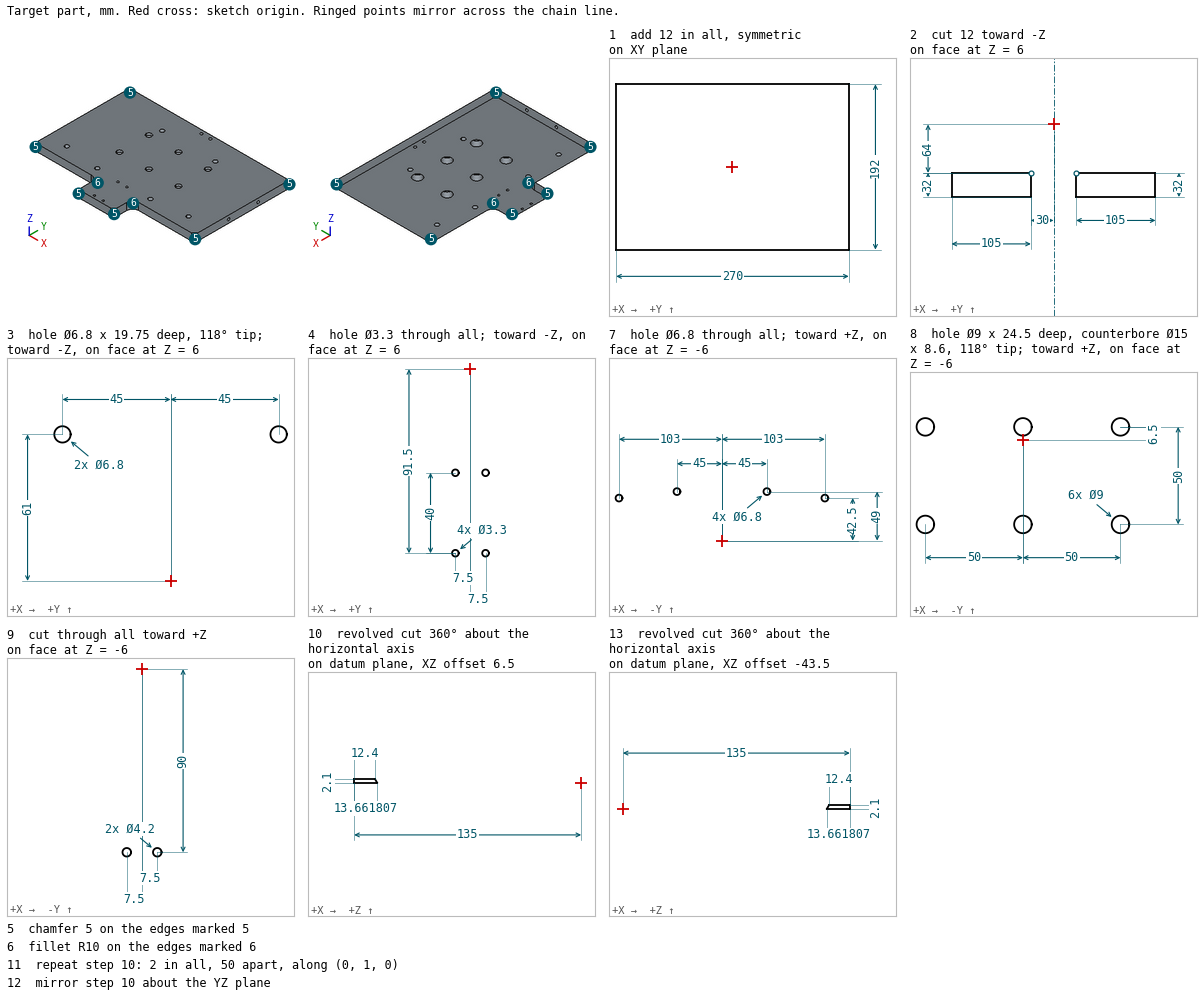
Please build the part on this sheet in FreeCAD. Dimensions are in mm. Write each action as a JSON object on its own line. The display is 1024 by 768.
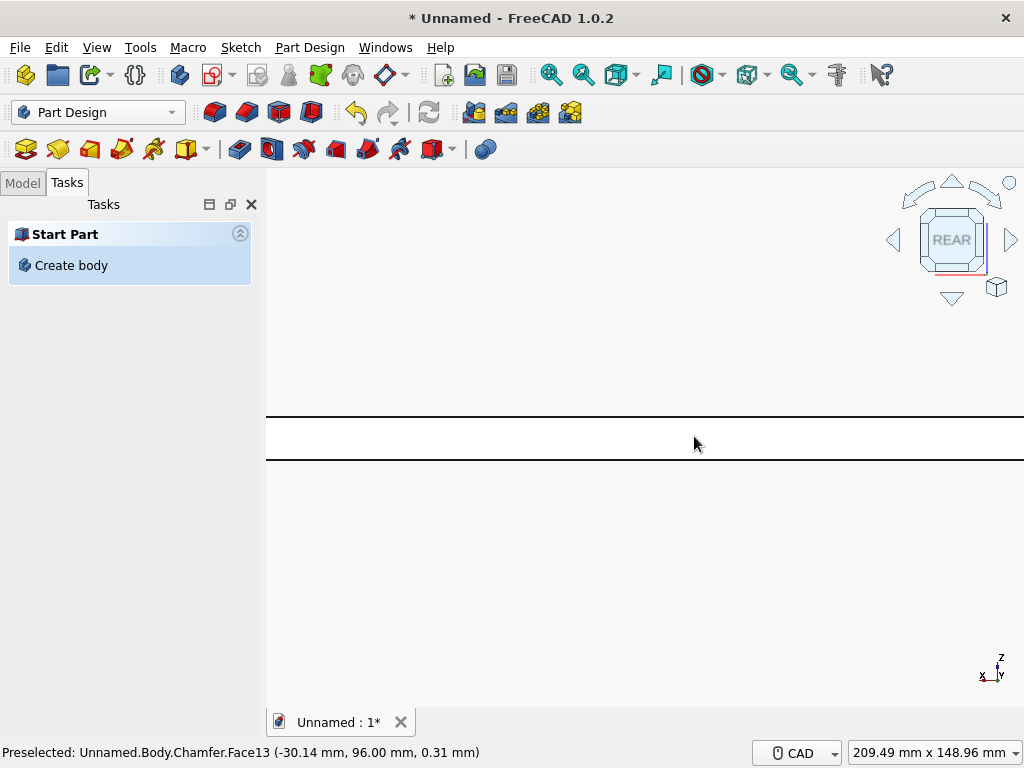
{"action": "key", "text": "v f"}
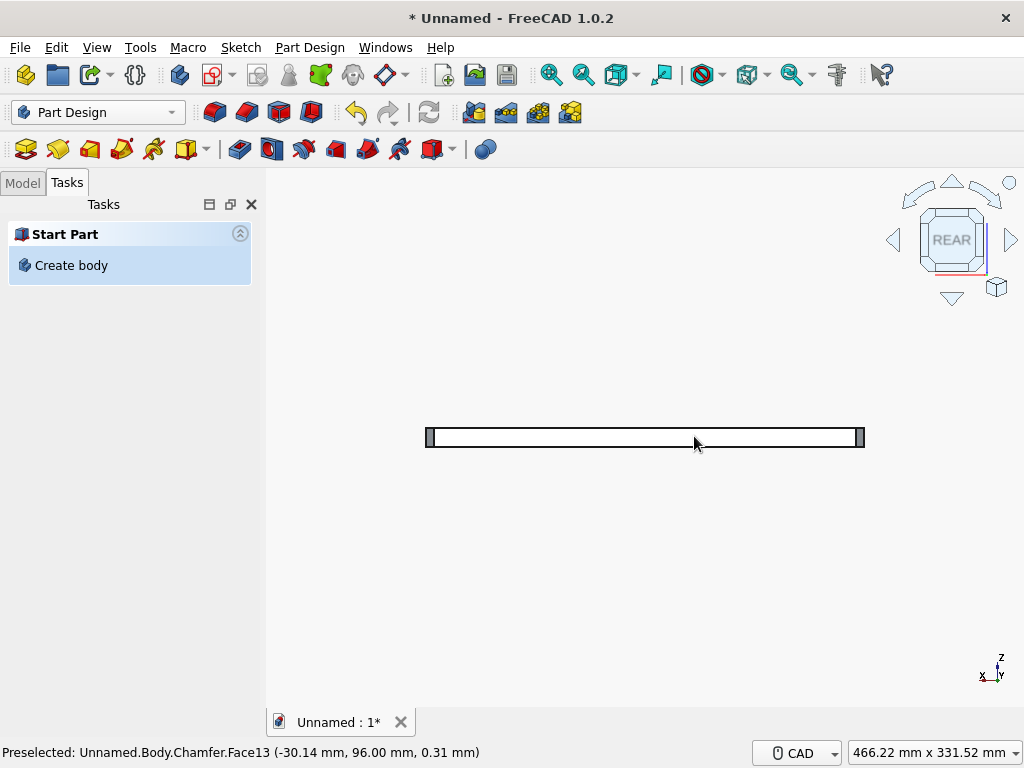
{"action": "key", "text": "0"}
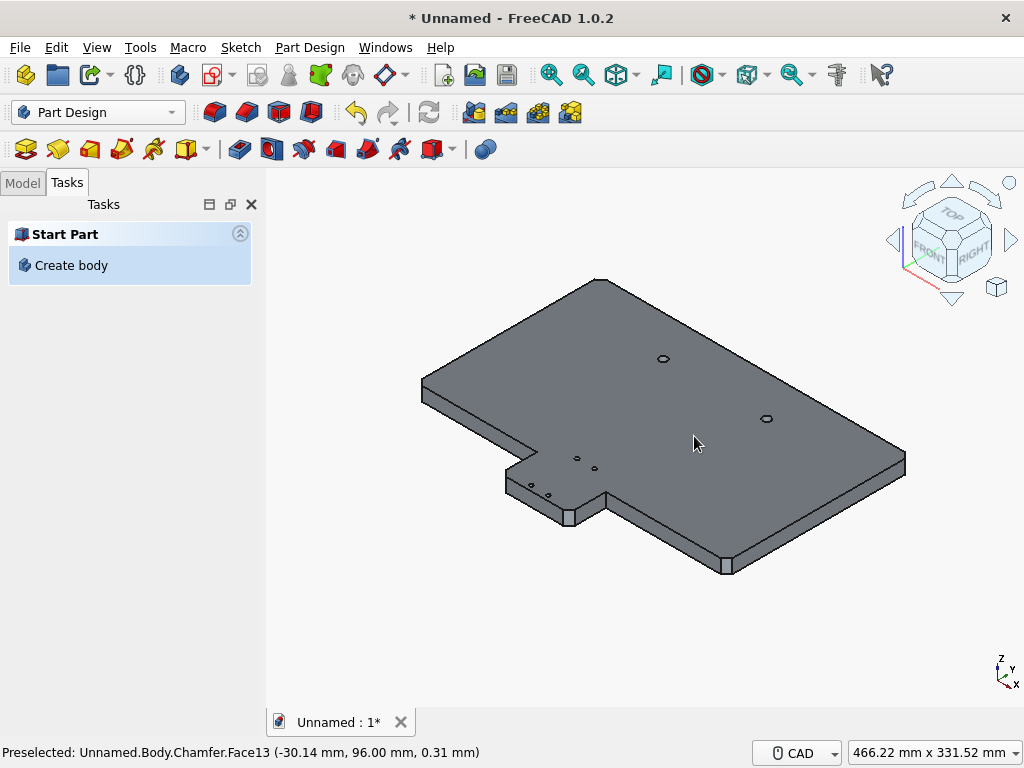
{"action": "scroll", "coordinate": [537, 459], "scroll_direction": "up", "scroll_amount": 4}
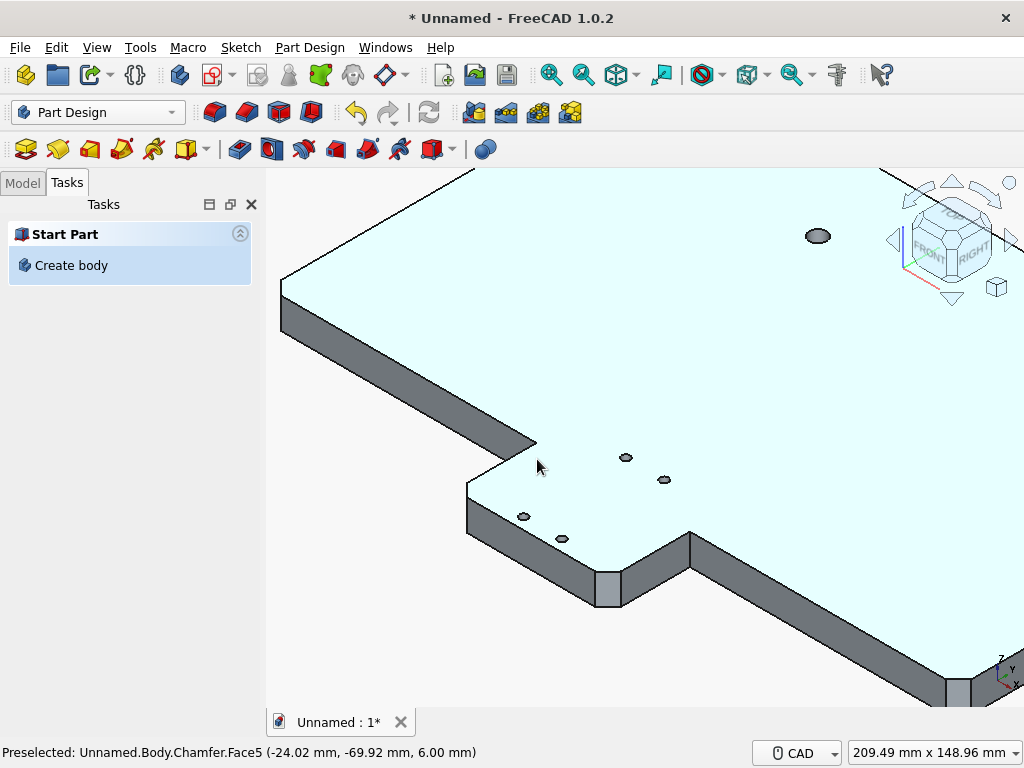
{"action": "key", "text": "v f"}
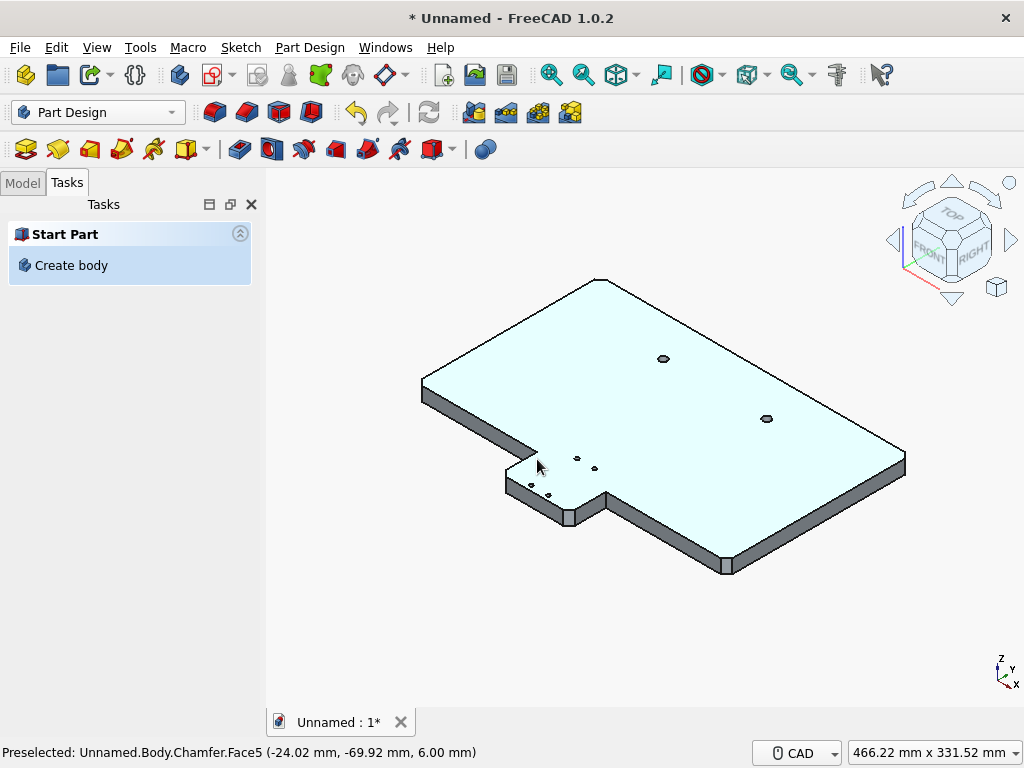
{"action": "key", "text": "2"}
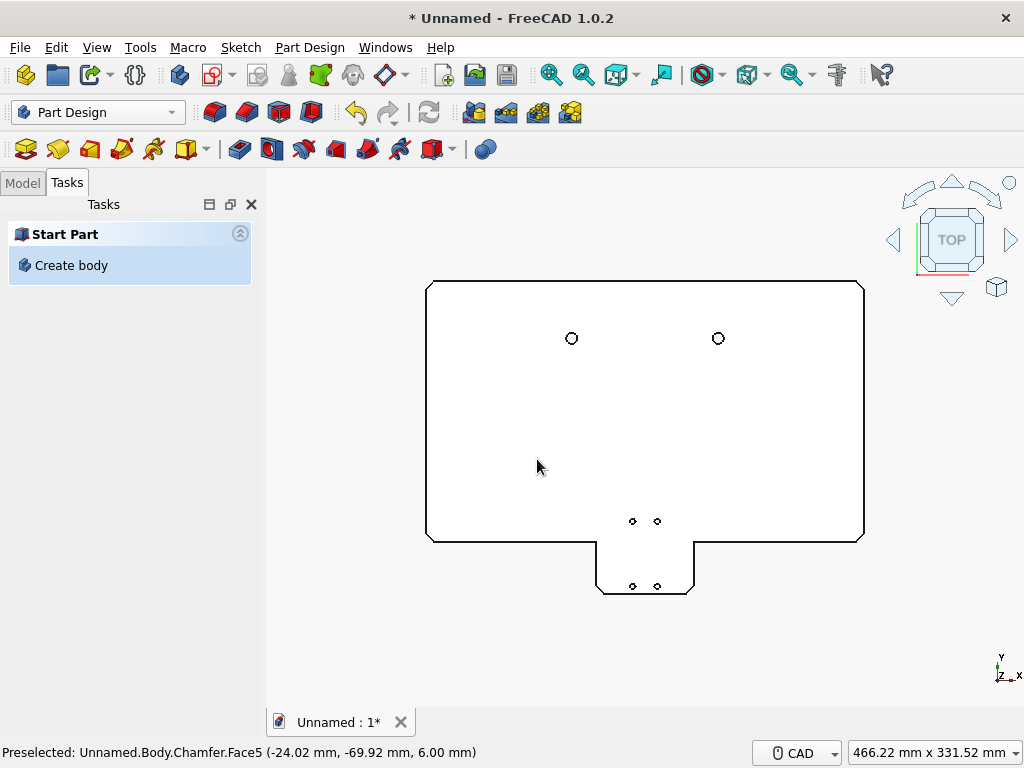
{"action": "scroll", "coordinate": [596, 541], "scroll_direction": "up", "scroll_amount": 4}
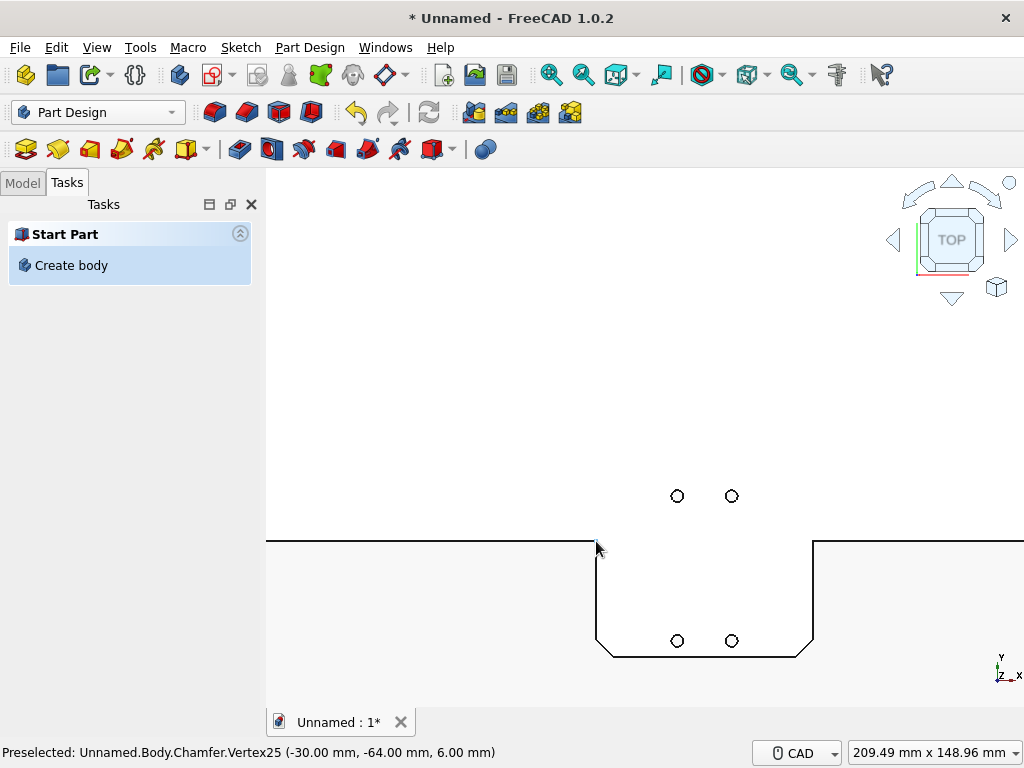
{"action": "left_click", "coordinate": [552, 76]}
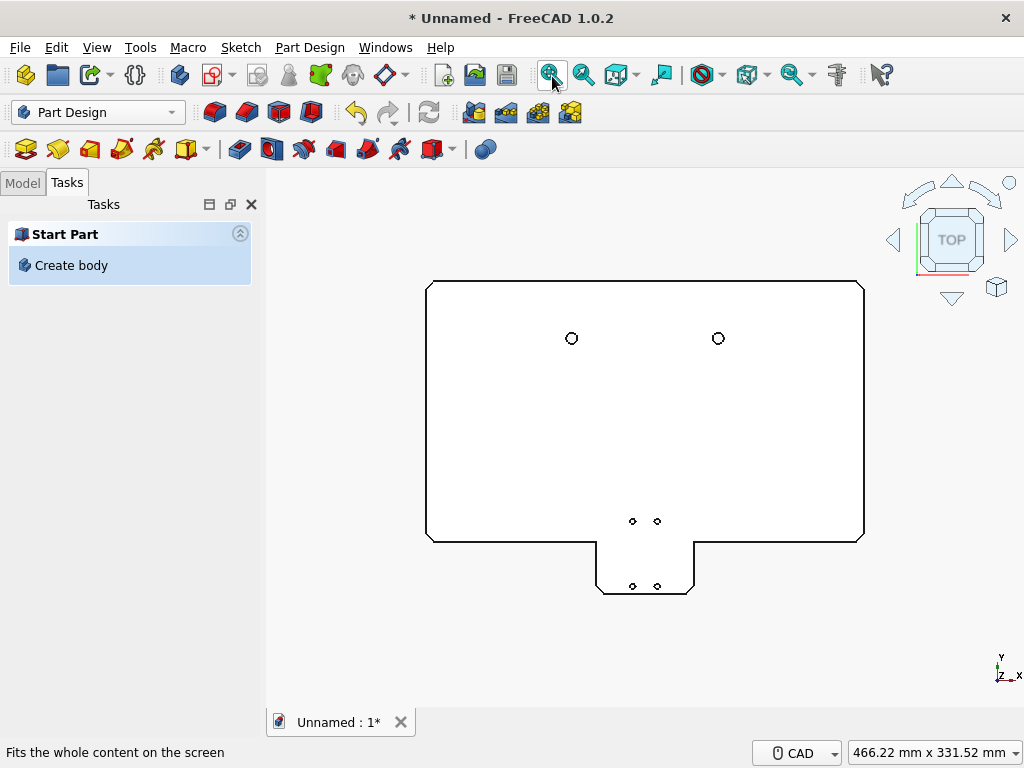
{"action": "key", "text": "1"}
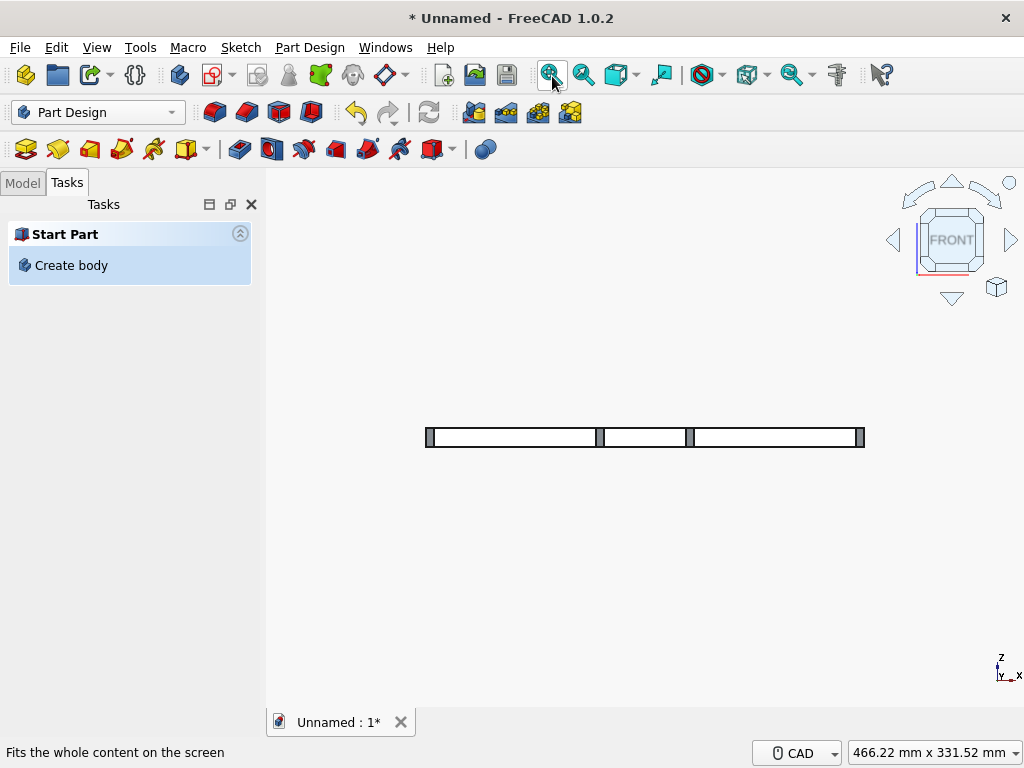
{"action": "scroll", "coordinate": [596, 436], "scroll_direction": "up", "scroll_amount": 4}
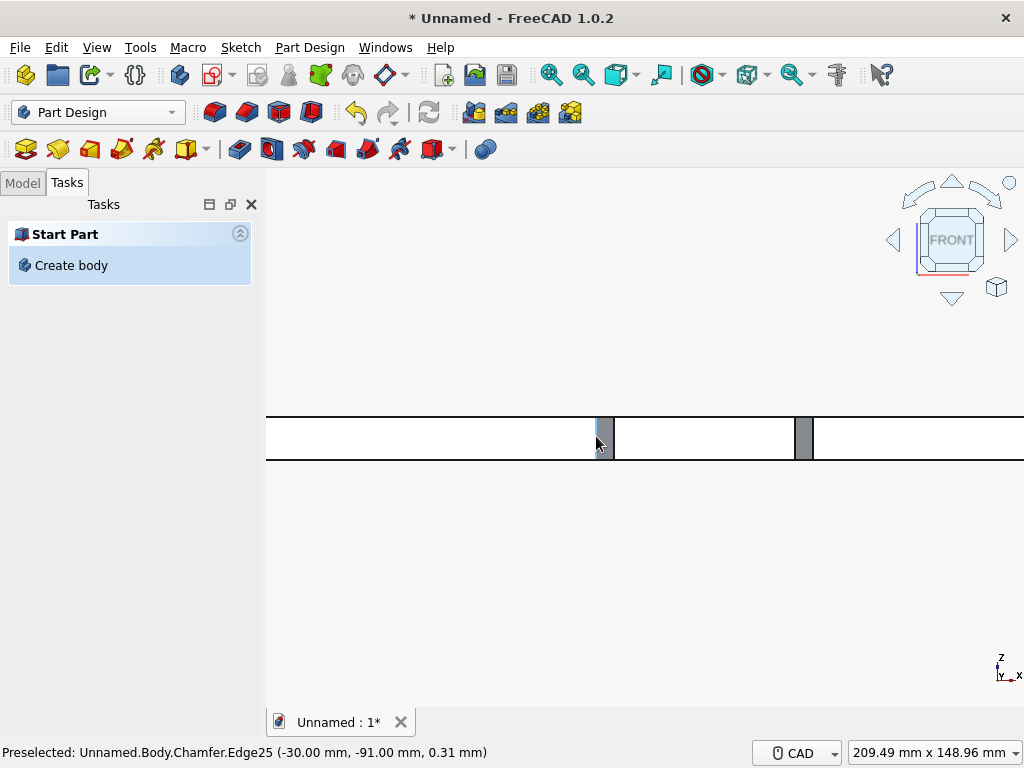
{"action": "key", "text": "v f"}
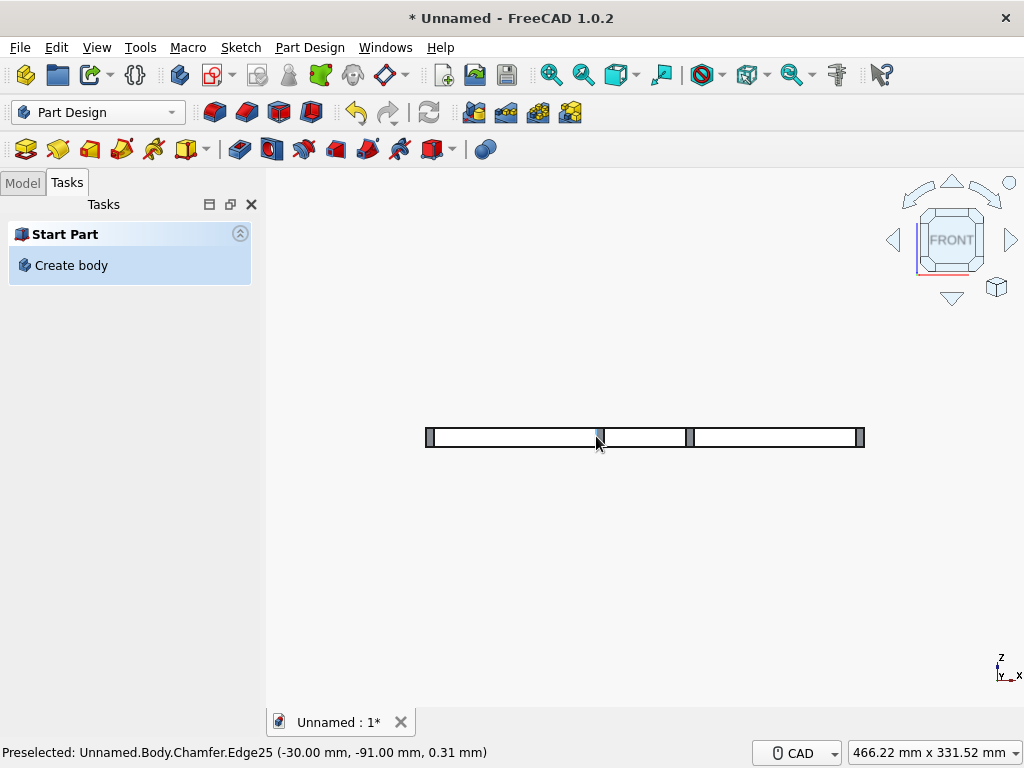
{"action": "key", "text": "3"}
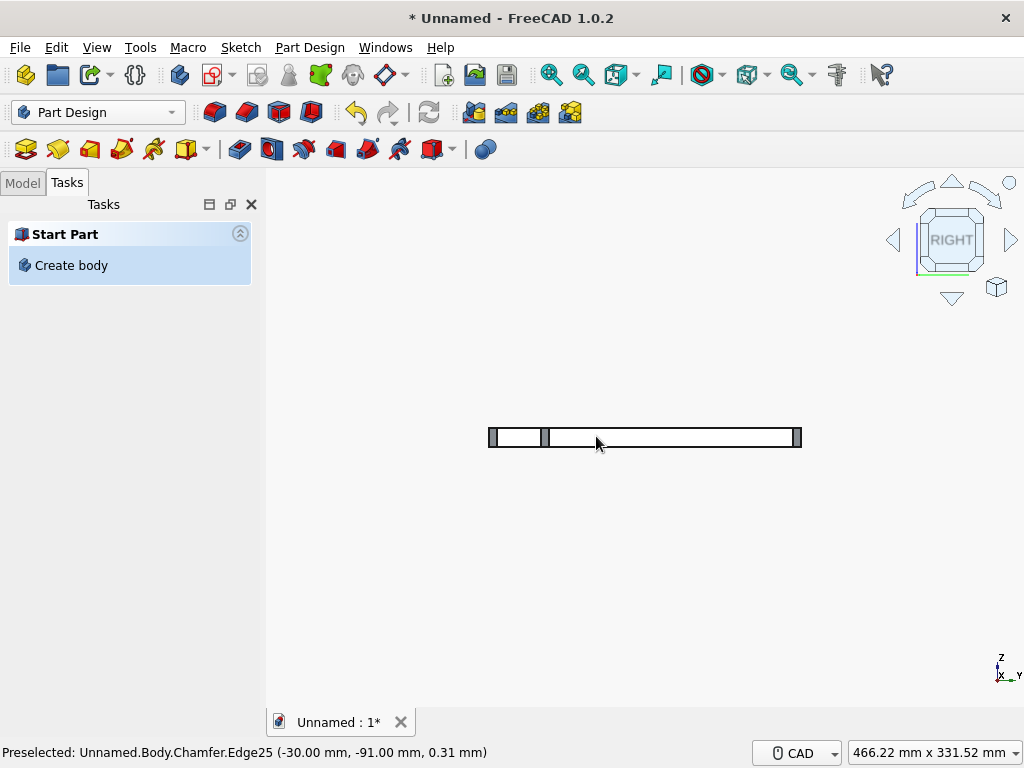
{"action": "key", "text": "v f"}